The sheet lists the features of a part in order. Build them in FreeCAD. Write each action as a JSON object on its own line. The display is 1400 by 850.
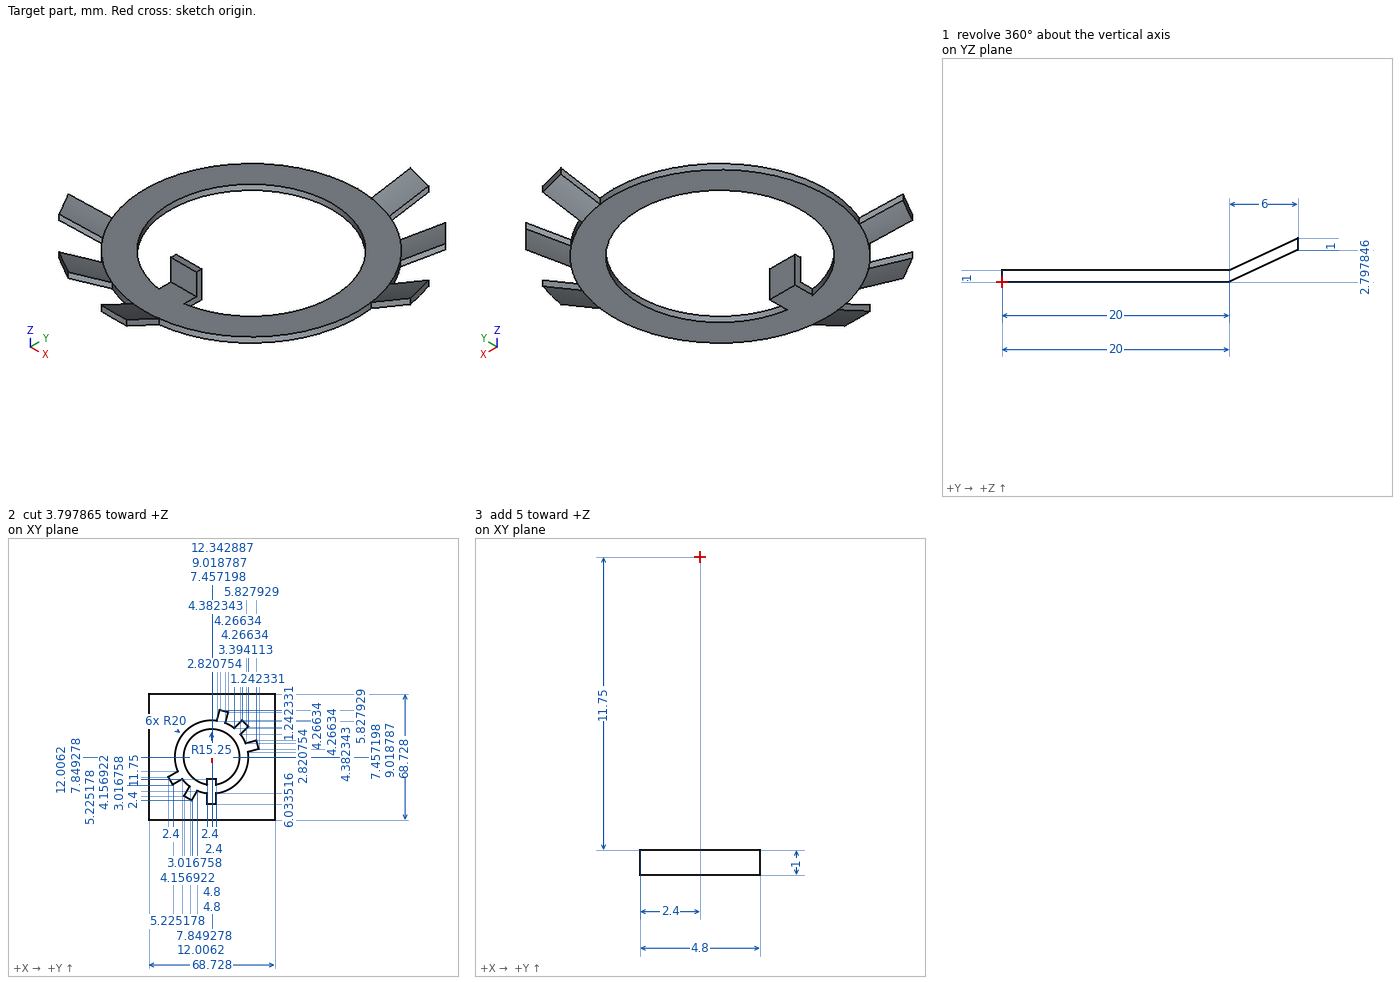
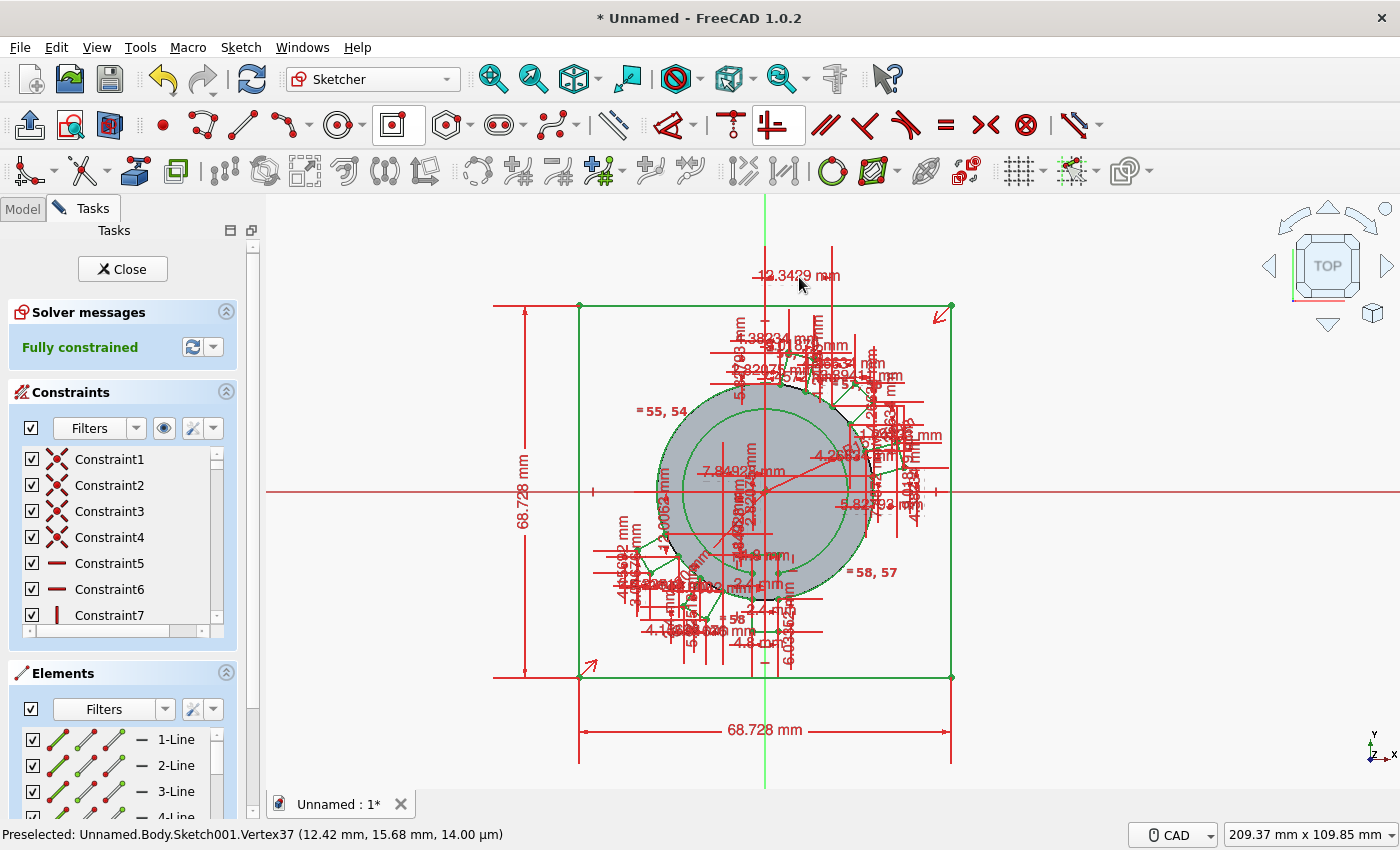
{"action": "left_click", "coordinate": [123, 269]}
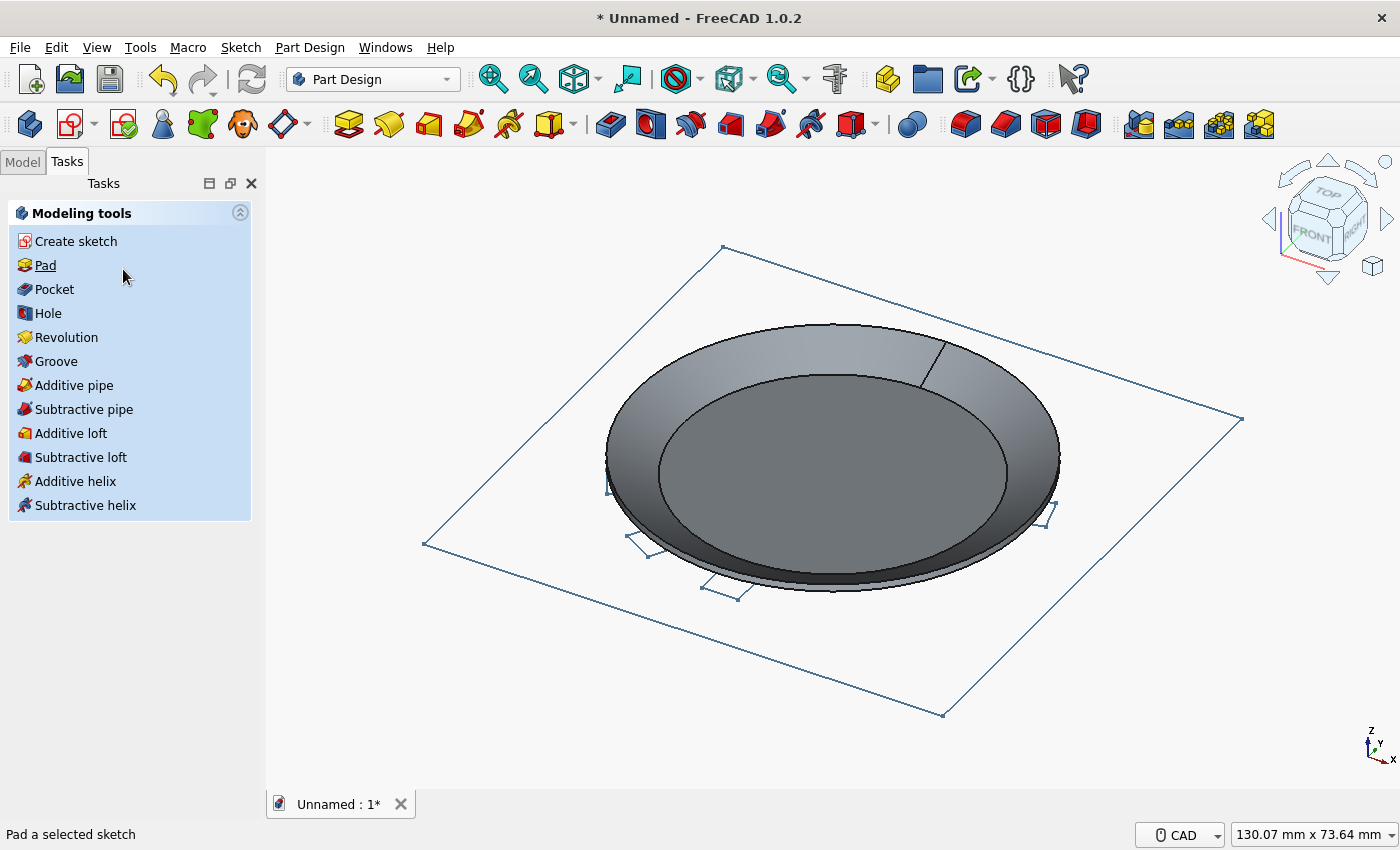
{"action": "left_click", "coordinate": [612, 124]}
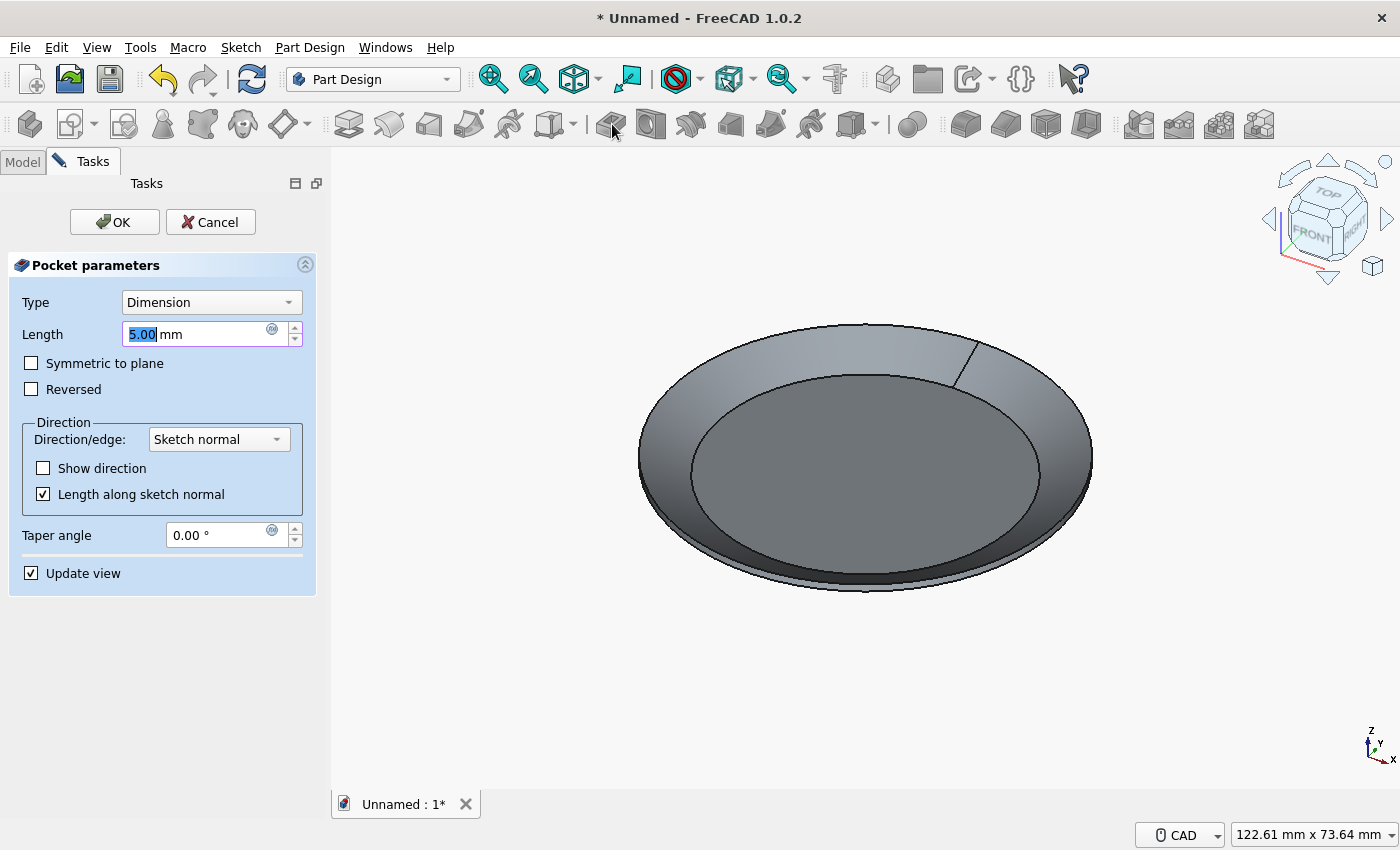
{"action": "type", "text": "3.797865"}
{"action": "key", "text": "Tab"}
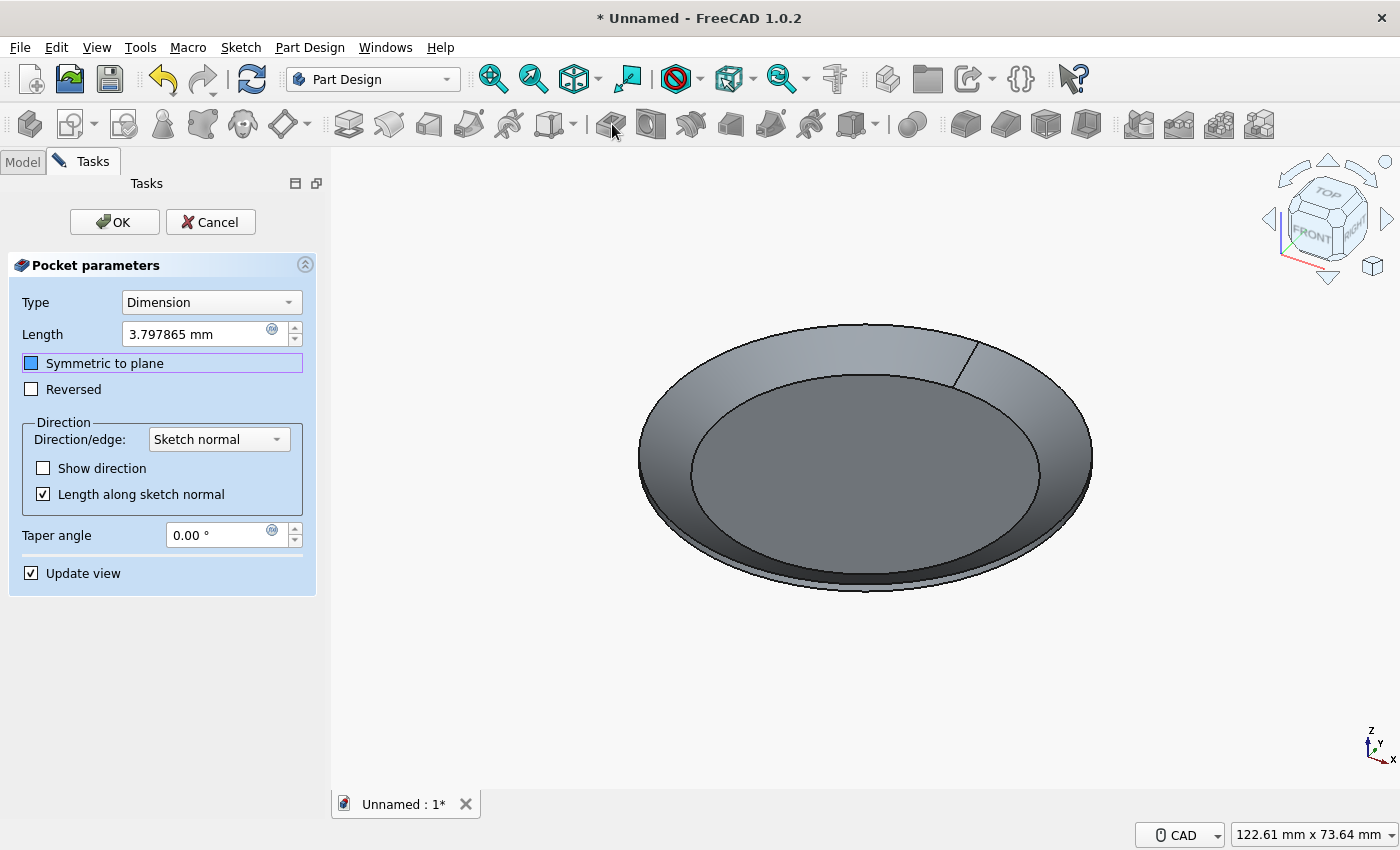
{"action": "left_click", "coordinate": [30, 389]}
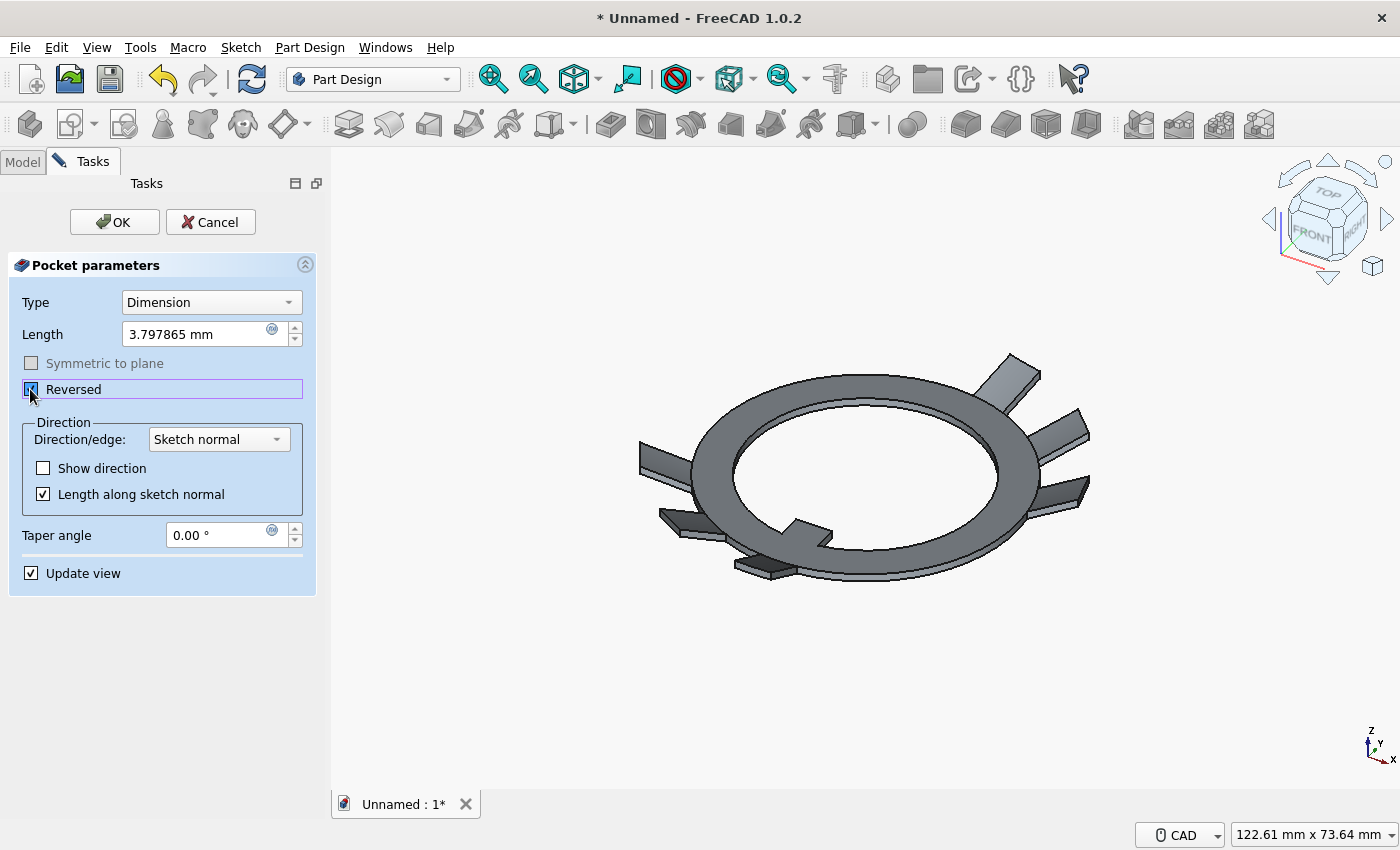
{"action": "left_click", "coordinate": [115, 222]}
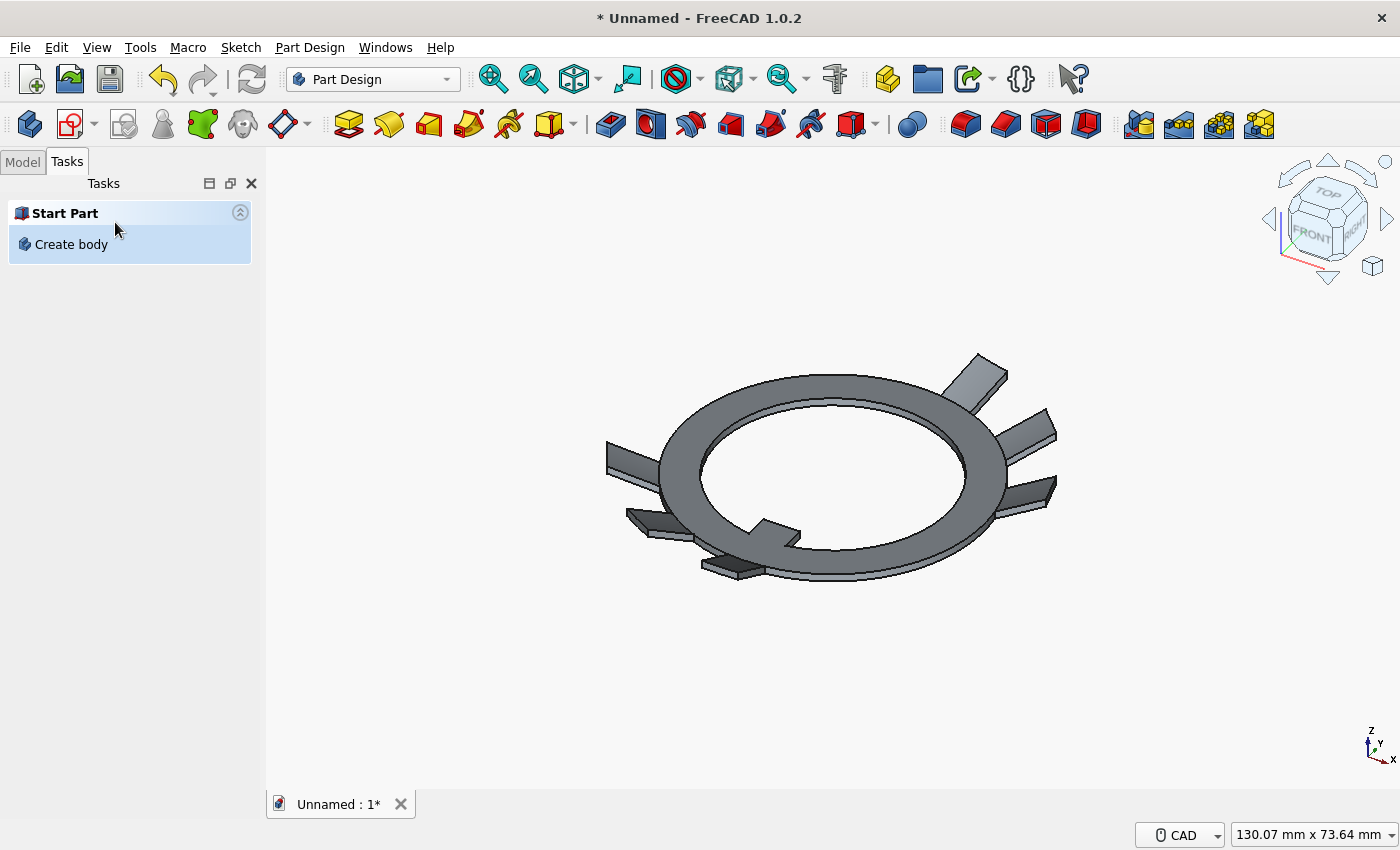
{"action": "left_click", "coordinate": [70, 124]}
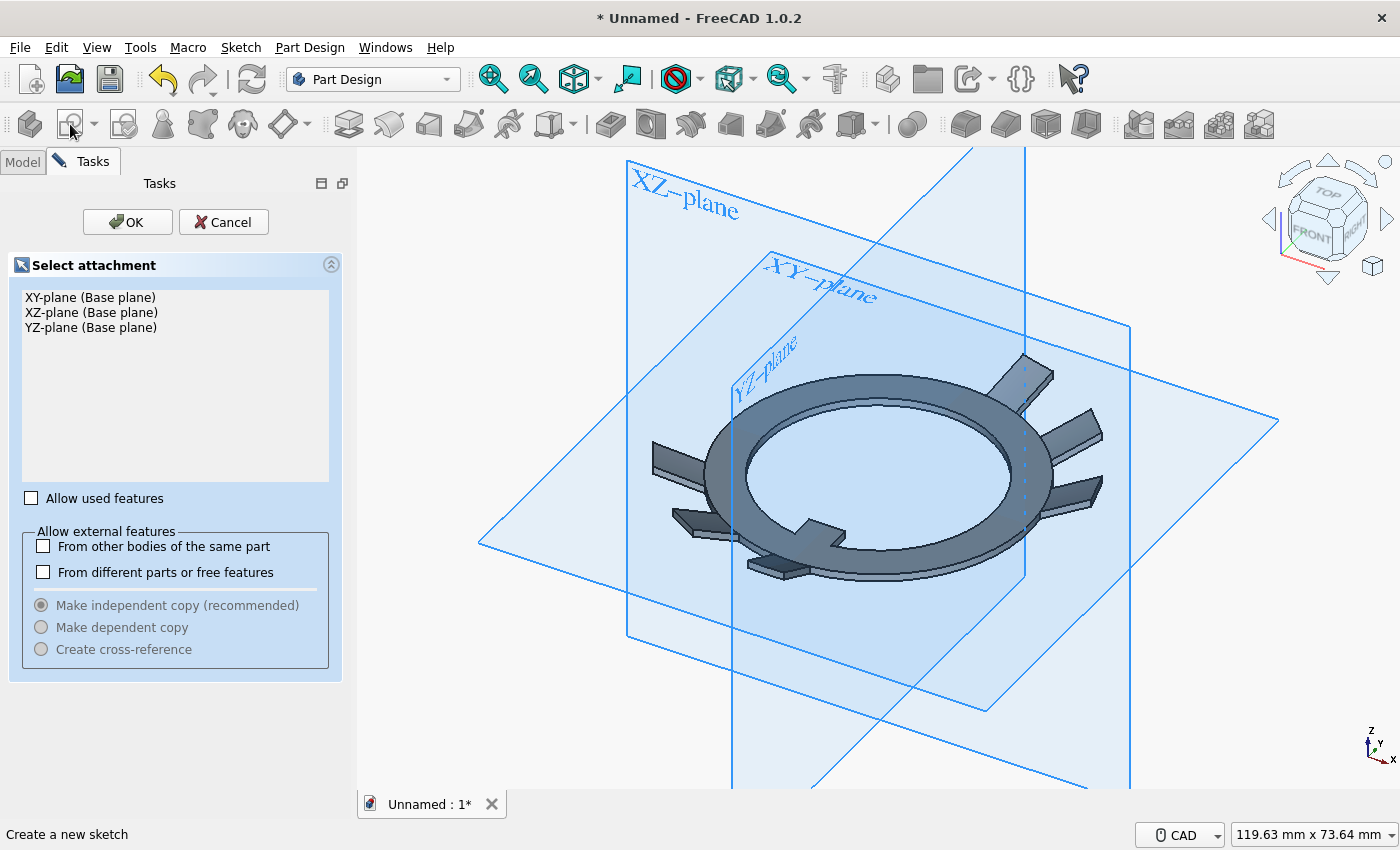
{"action": "left_click", "coordinate": [82, 298]}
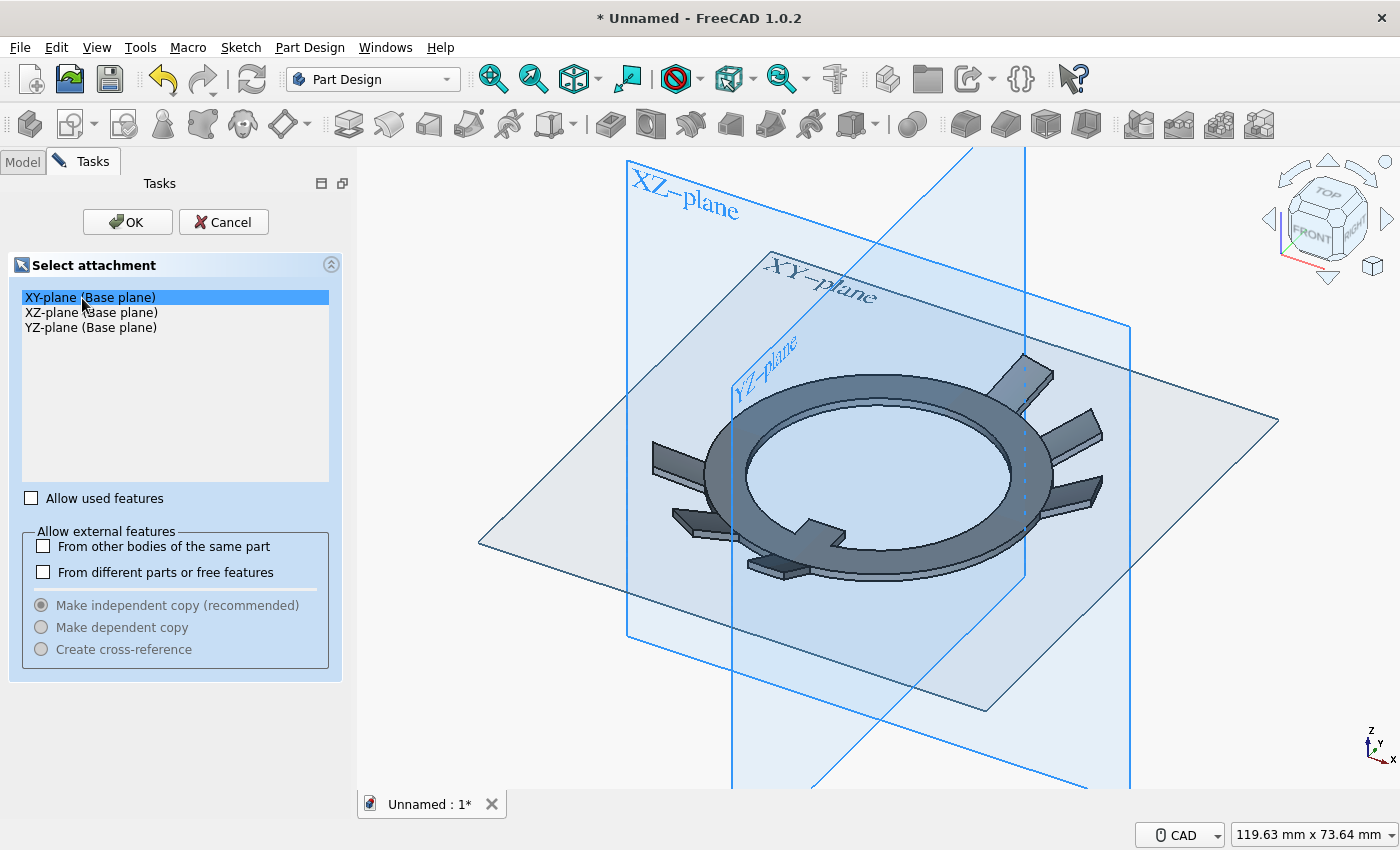
{"action": "left_click", "coordinate": [128, 222]}